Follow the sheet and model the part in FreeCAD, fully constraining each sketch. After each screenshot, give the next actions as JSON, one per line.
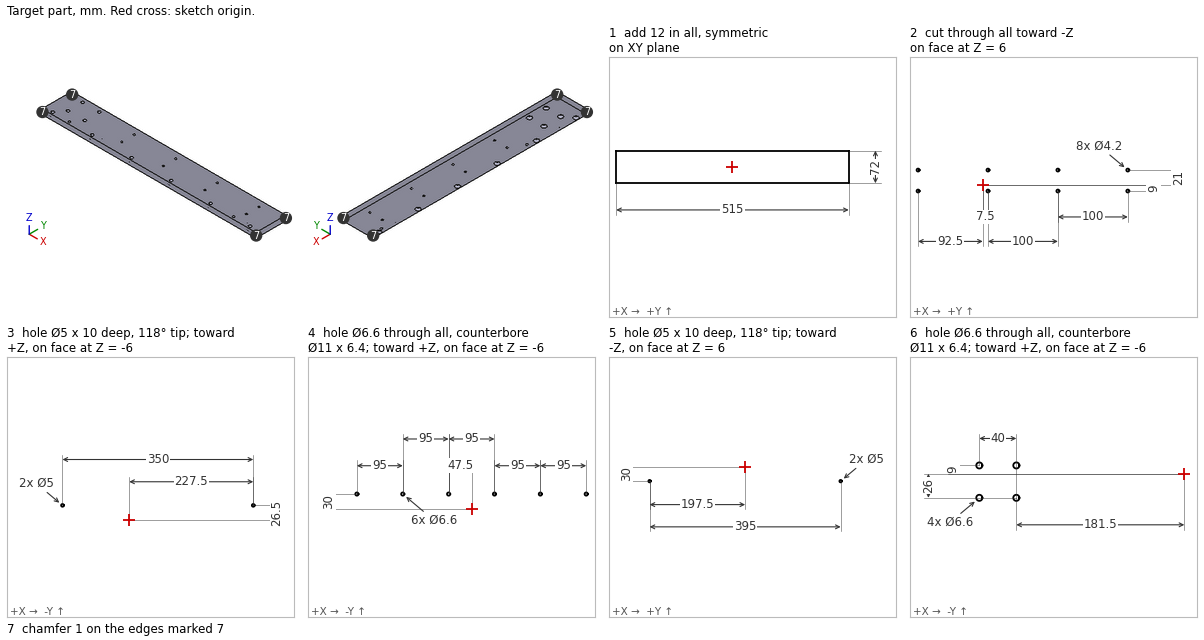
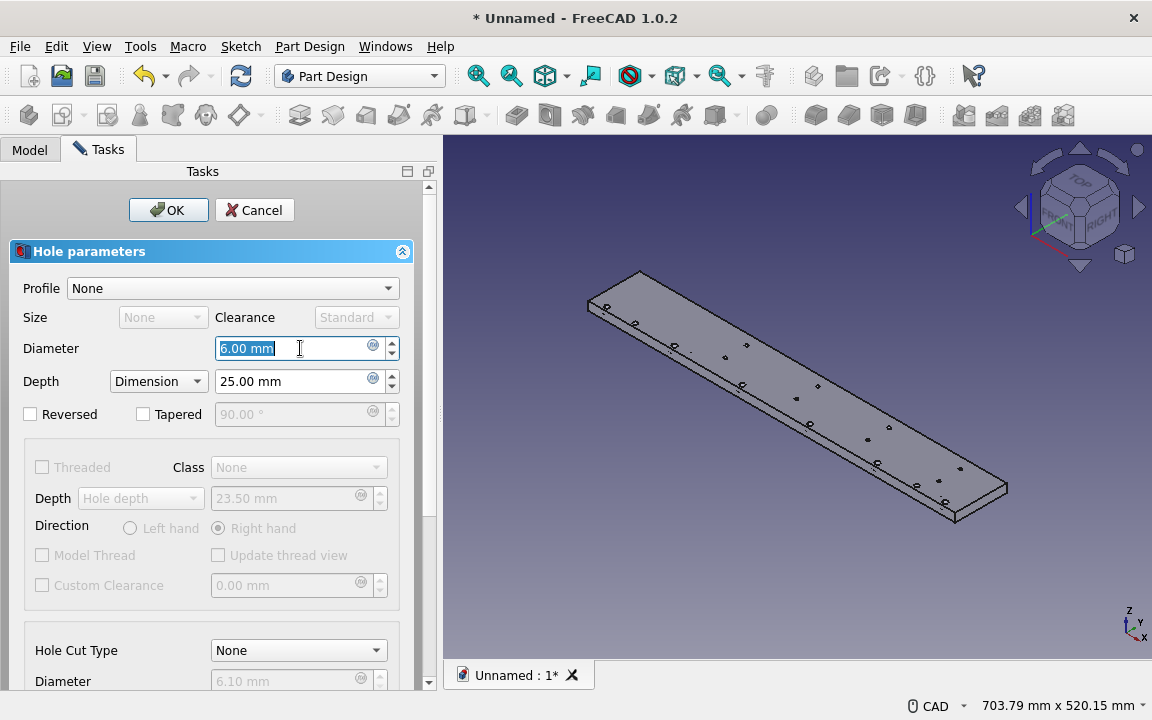
{"action": "type", "text": "5"}
{"action": "key", "text": "Tab"}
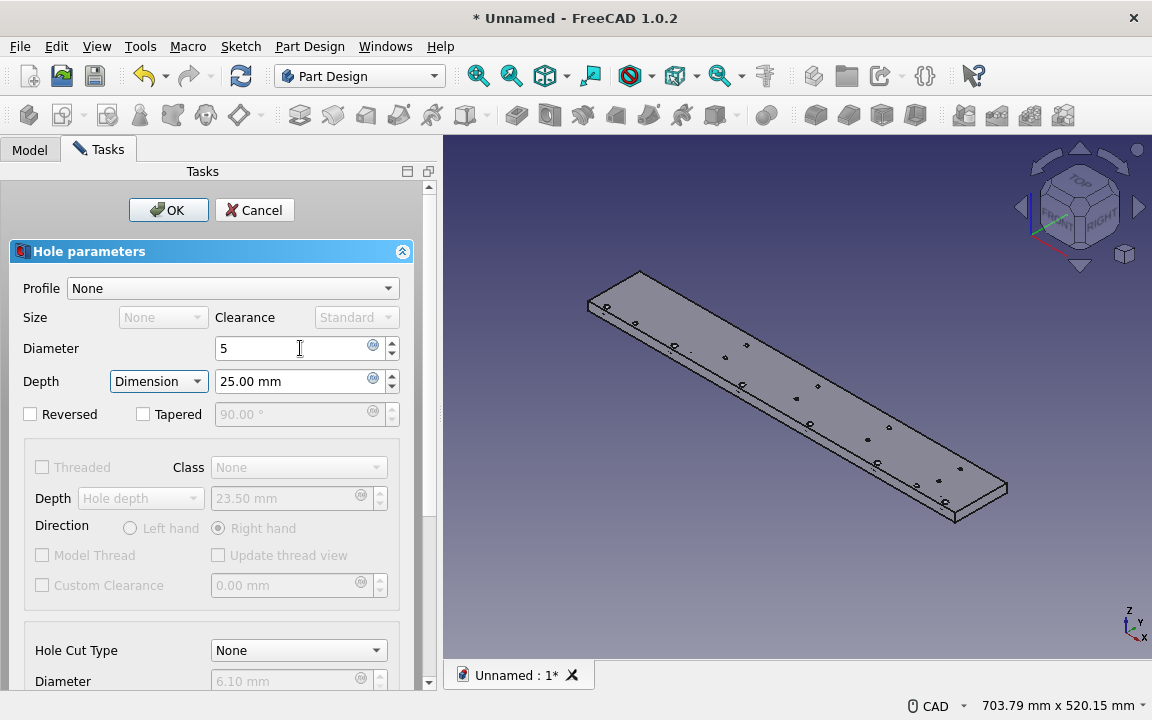
{"action": "triple_click", "coordinate": [300, 382]}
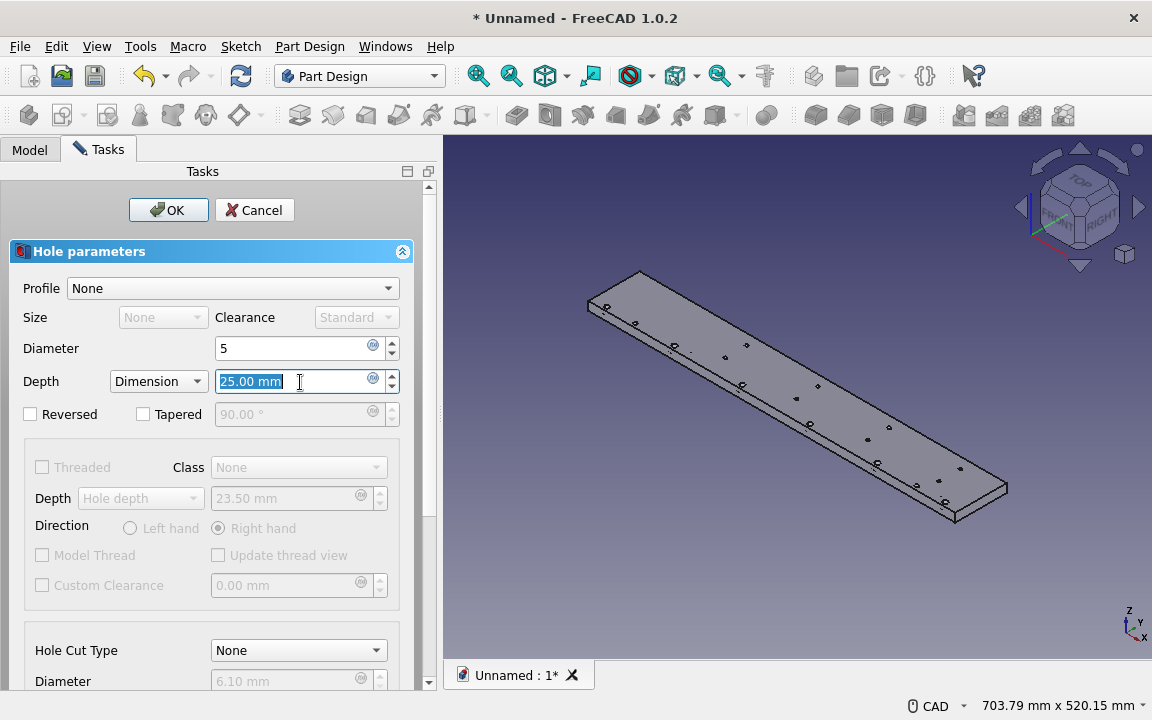
{"action": "type", "text": "10"}
{"action": "key", "text": "Tab"}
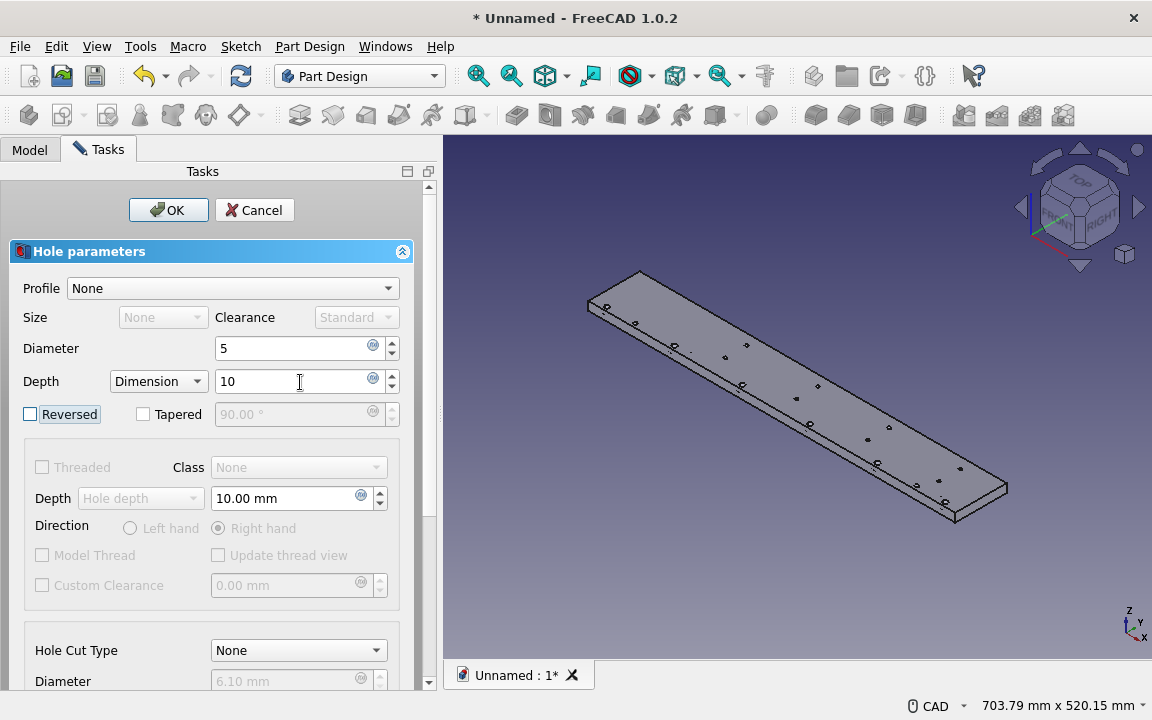
{"action": "left_click", "coordinate": [169, 210]}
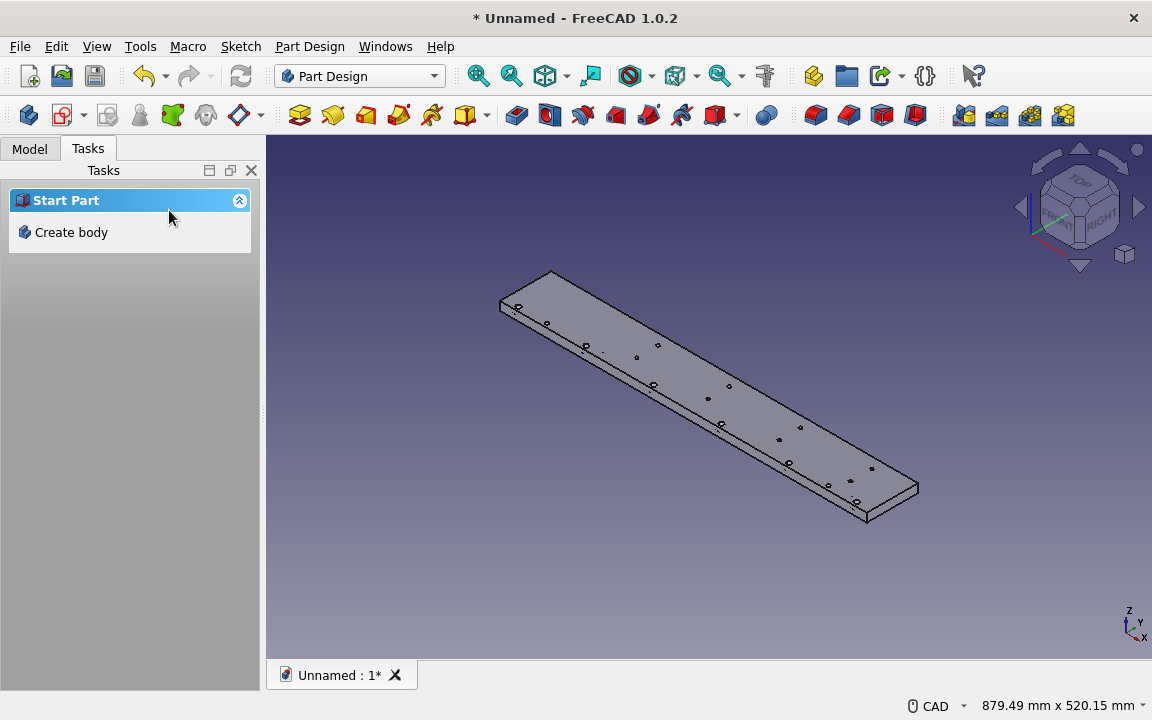
{"action": "key", "text": "5"}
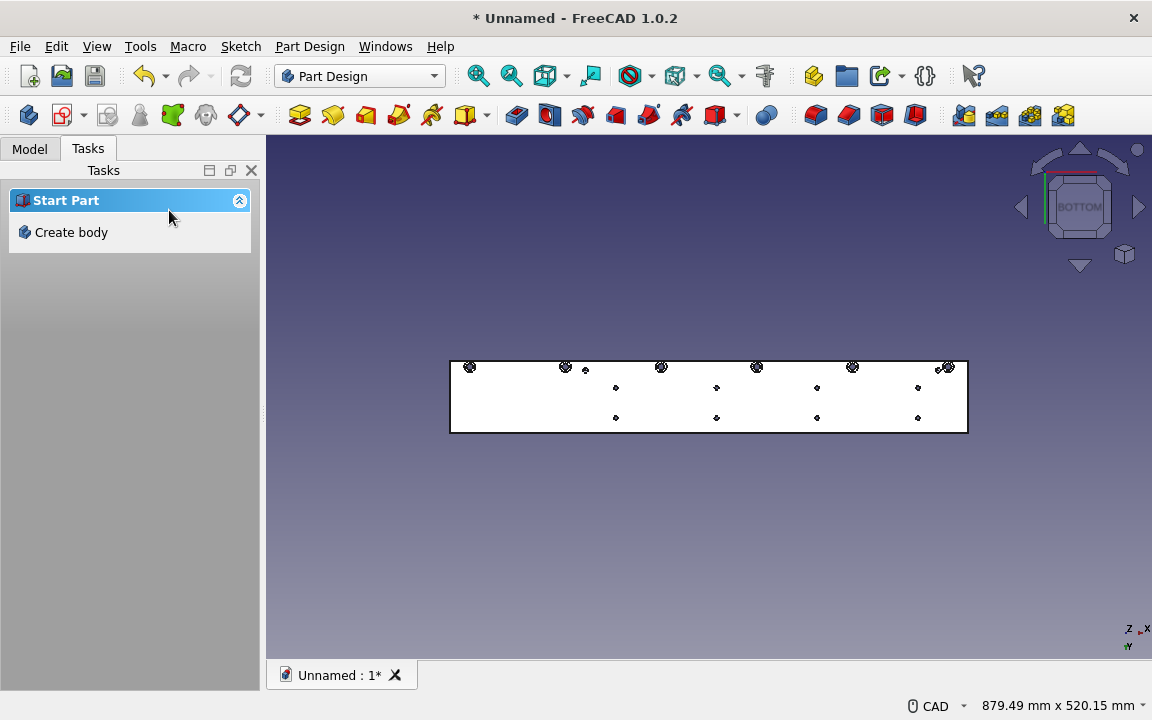
{"action": "left_click", "coordinate": [783, 396]}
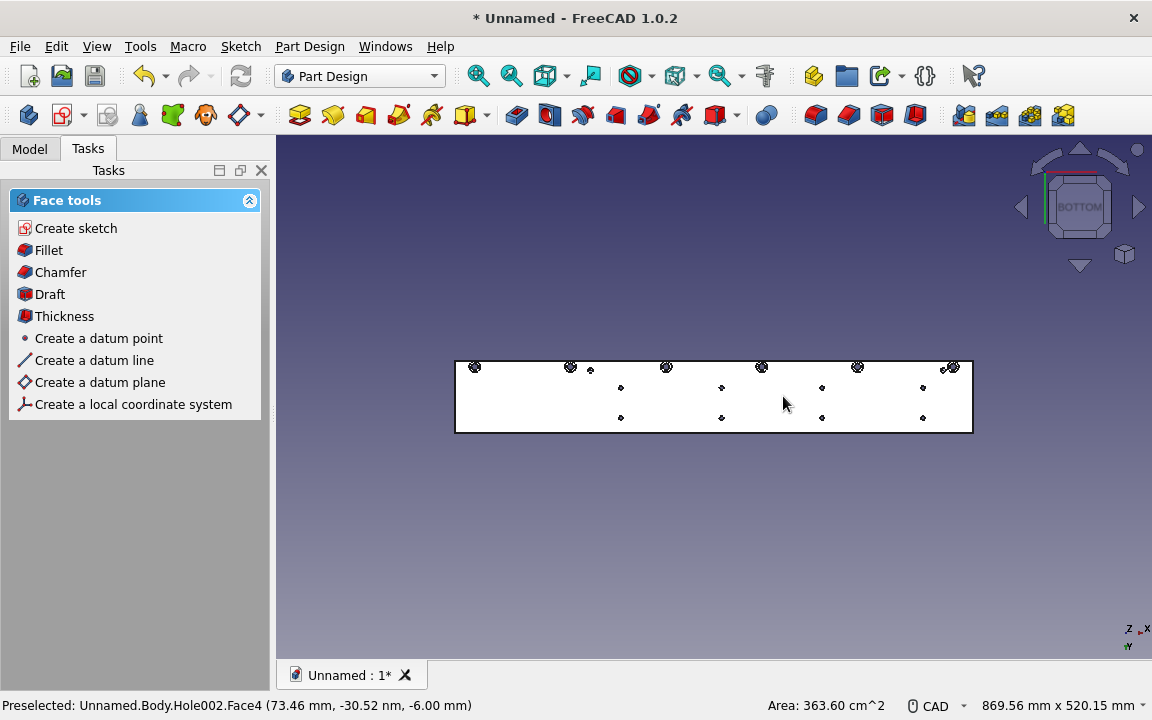
{"action": "left_click", "coordinate": [62, 116]}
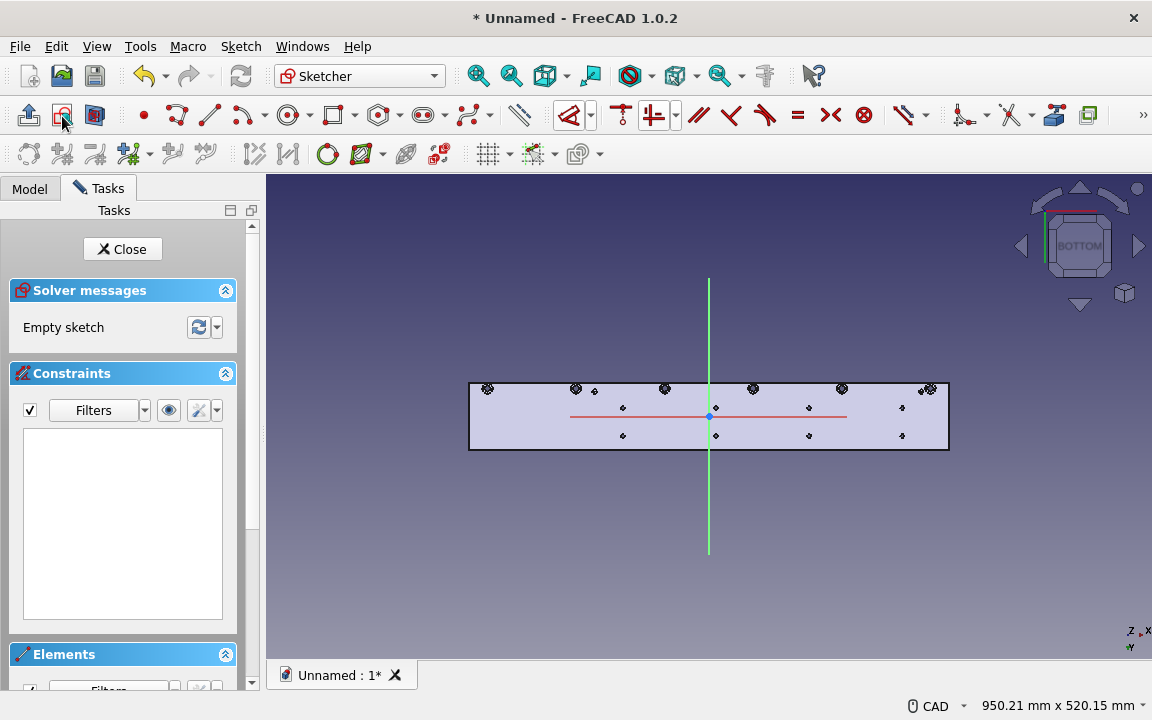
{"action": "scroll", "coordinate": [502, 426], "scroll_direction": "up", "scroll_amount": 10}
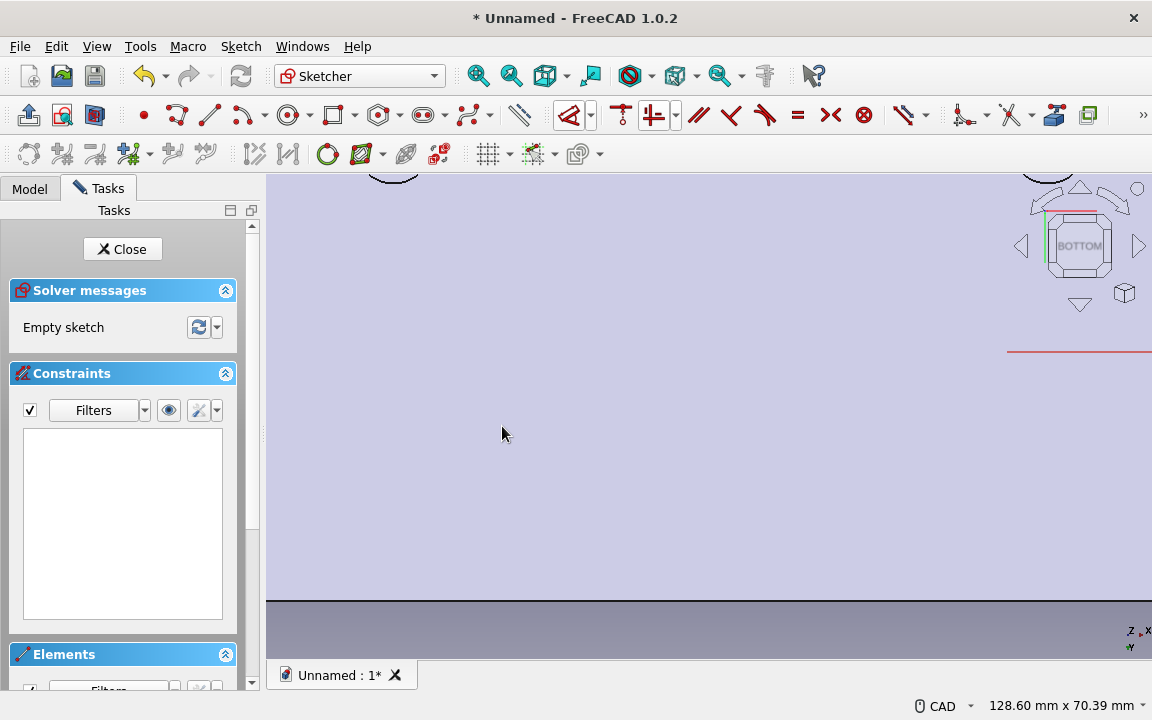
{"action": "left_click", "coordinate": [288, 116]}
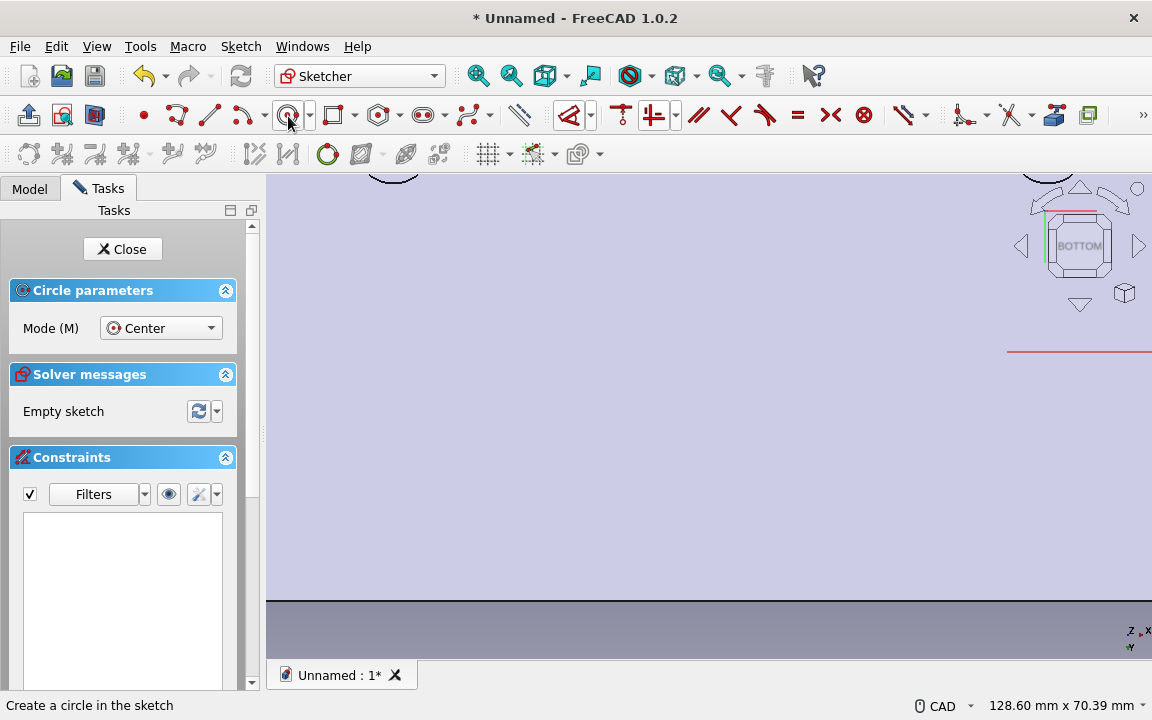
{"action": "left_click", "coordinate": [779, 532]}
{"action": "mouse_move", "coordinate": [795, 516]}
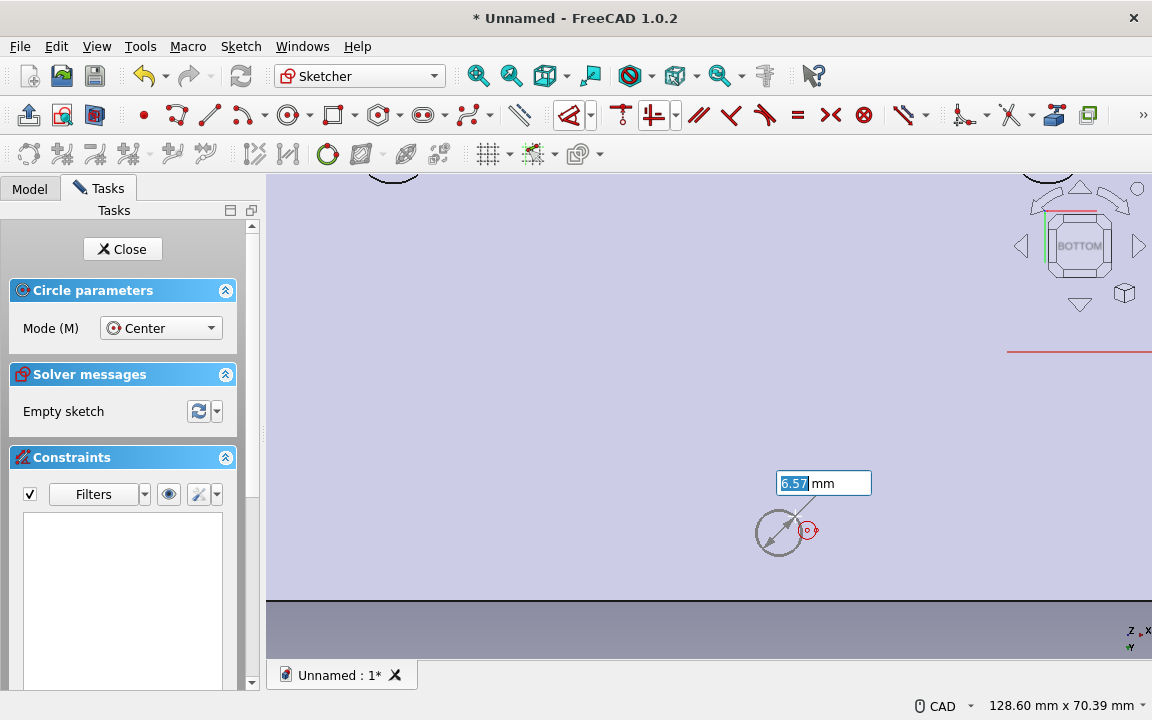
{"action": "type", "text": "6.6"}
{"action": "key", "text": "Return"}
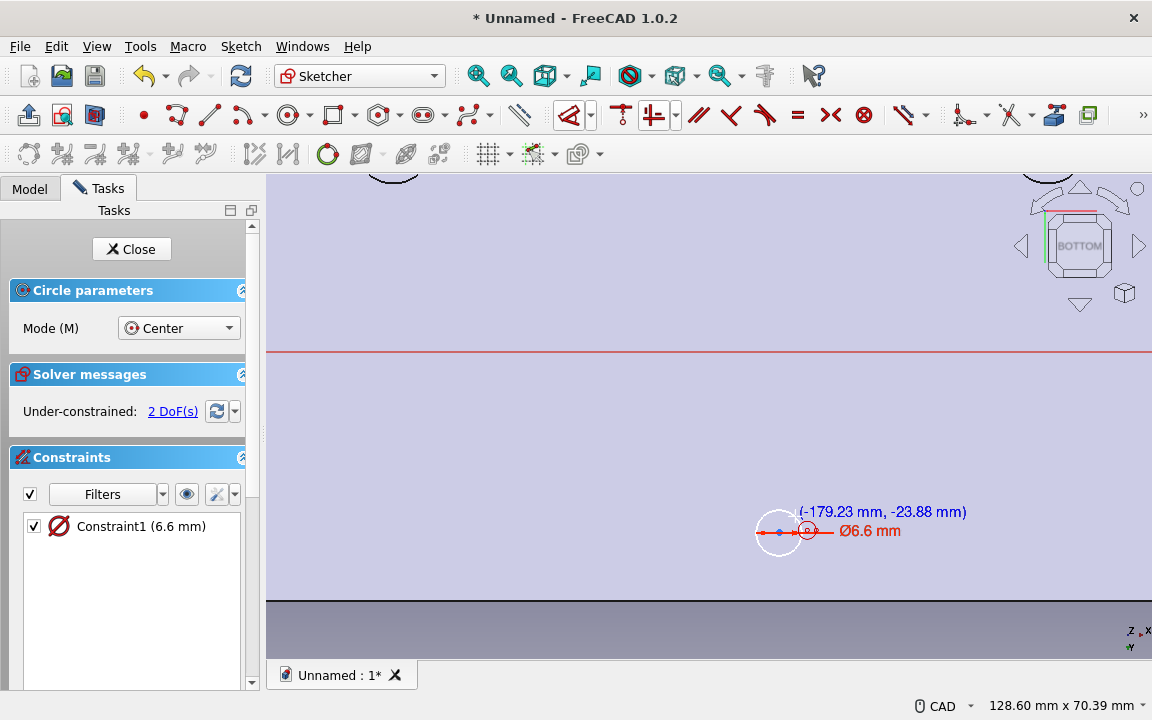
{"action": "left_click", "coordinate": [504, 290]}
{"action": "mouse_move", "coordinate": [520, 274]}